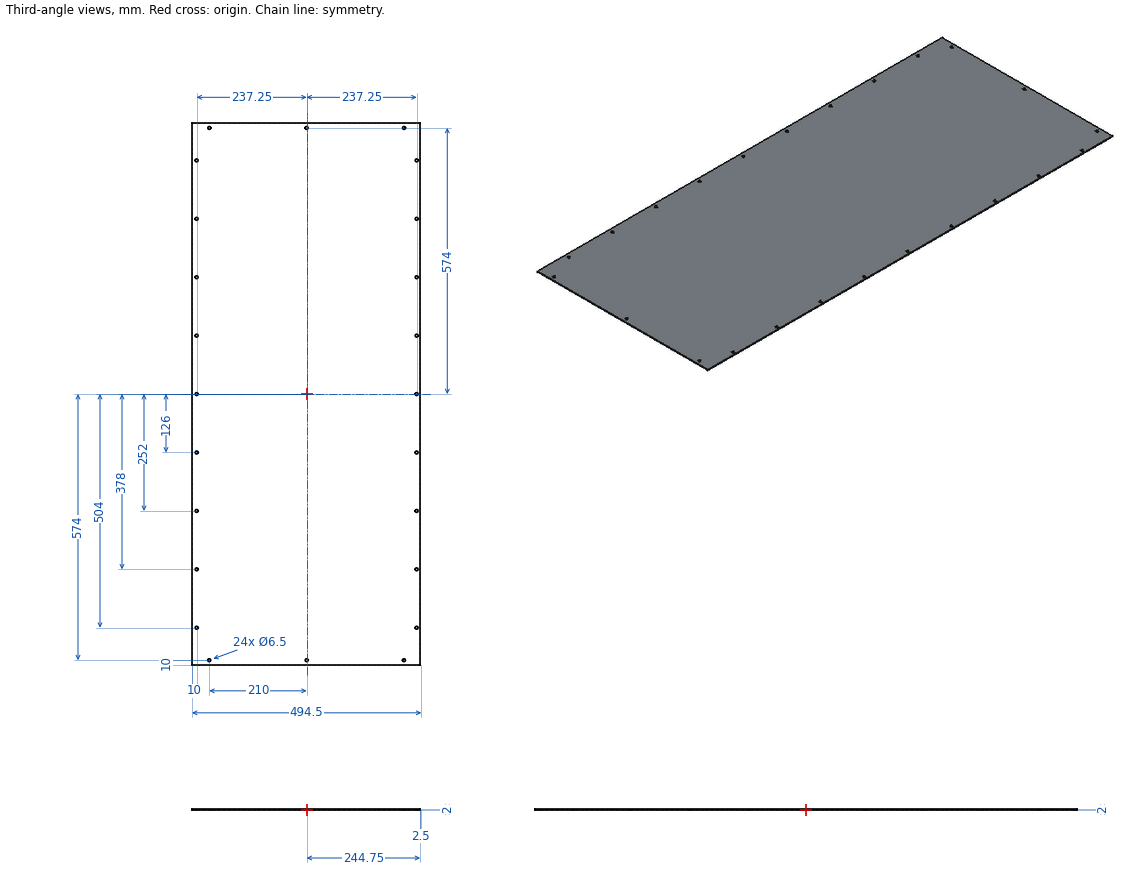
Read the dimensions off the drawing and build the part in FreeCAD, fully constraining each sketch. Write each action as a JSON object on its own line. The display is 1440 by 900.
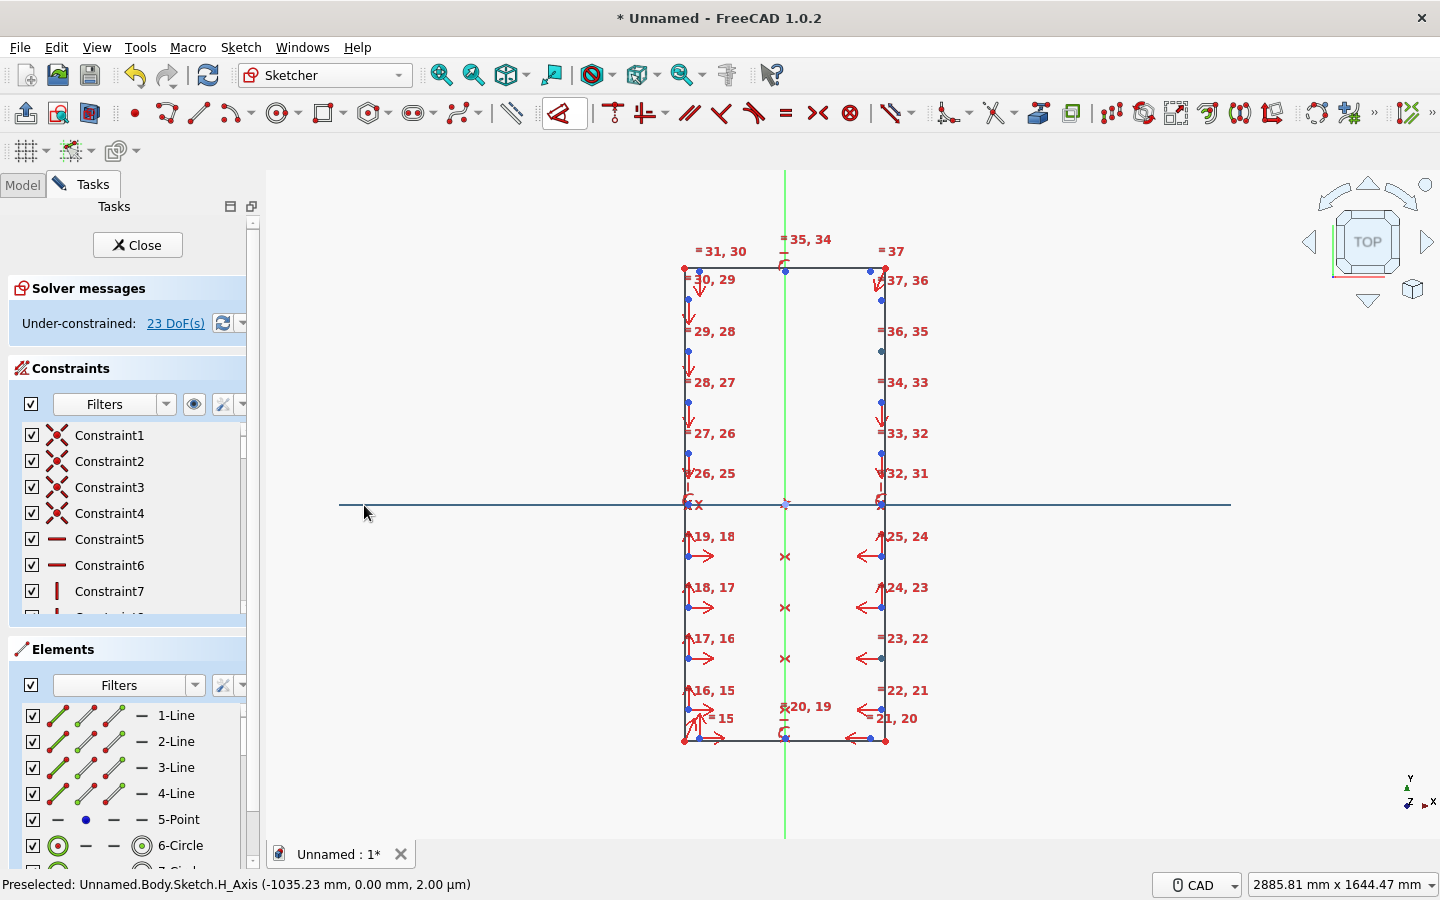
{"action": "key", "text": "s"}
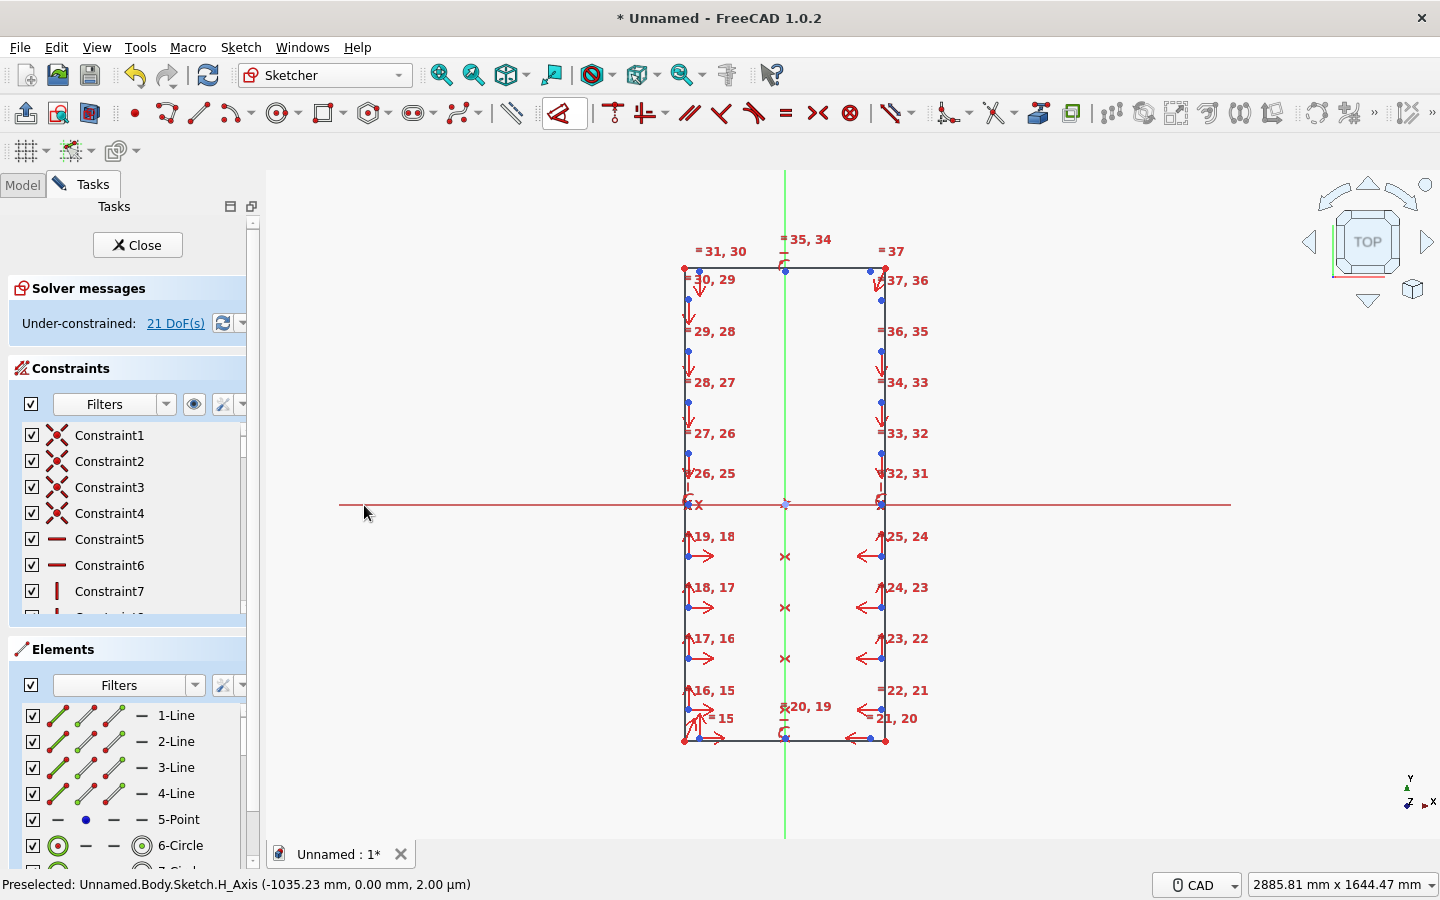
{"action": "left_click", "coordinate": [882, 710]}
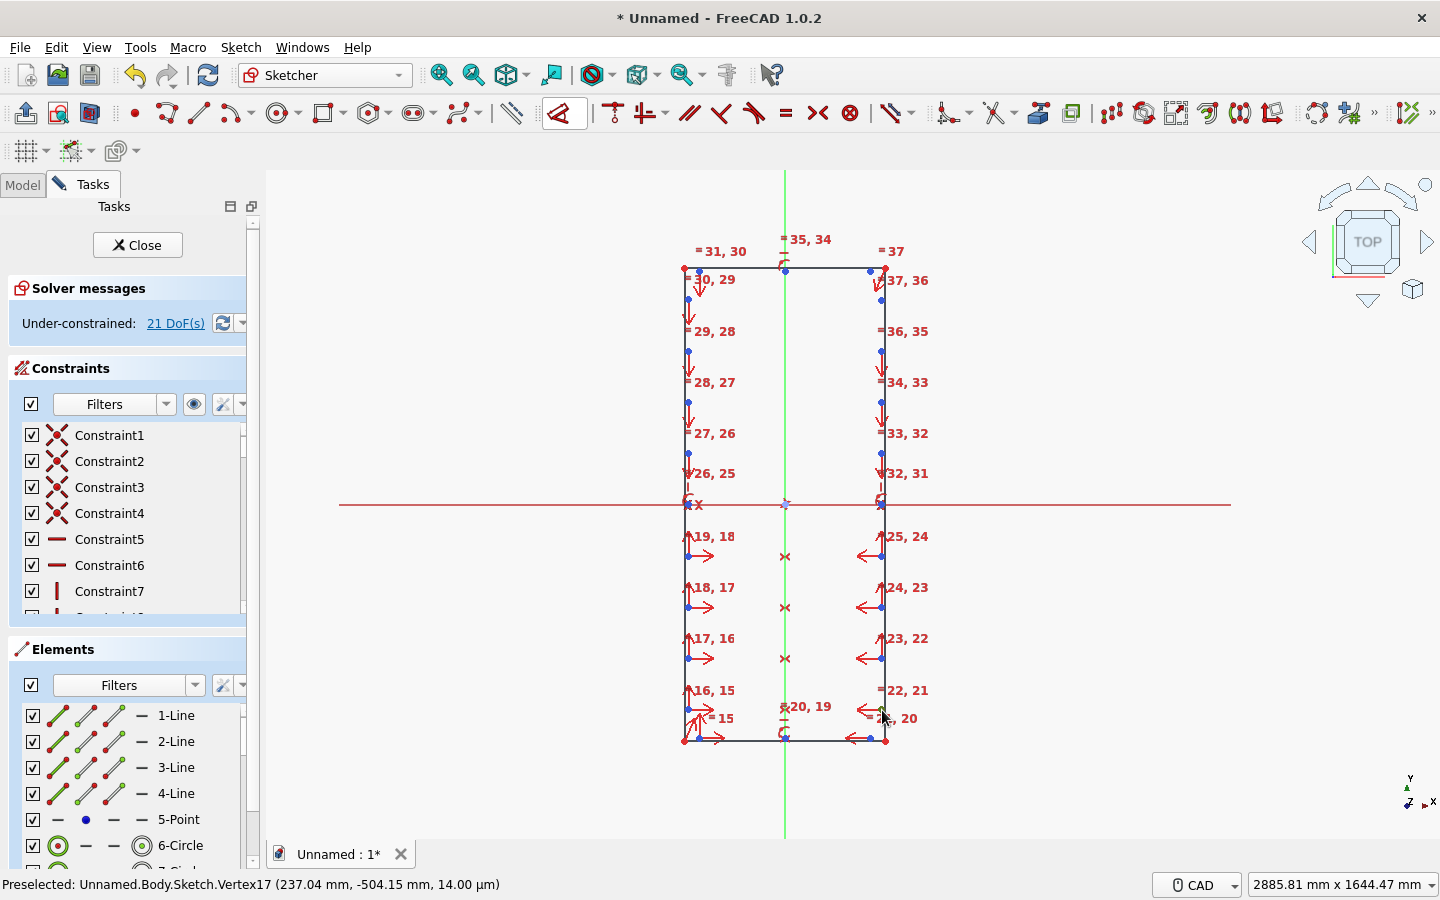
{"action": "left_click", "coordinate": [882, 300]}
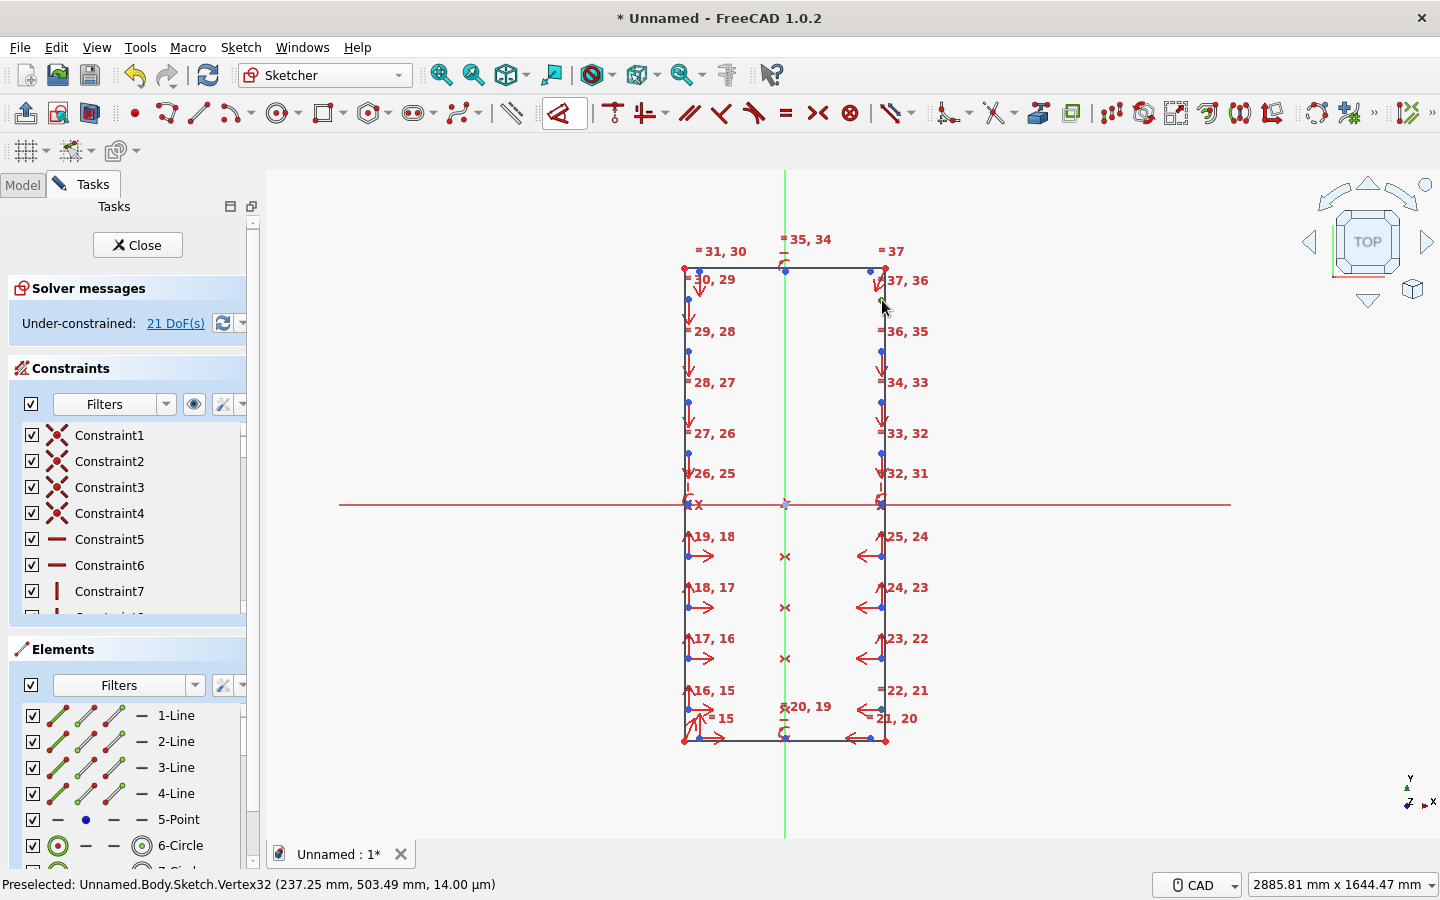
{"action": "left_click", "coordinate": [364, 505]}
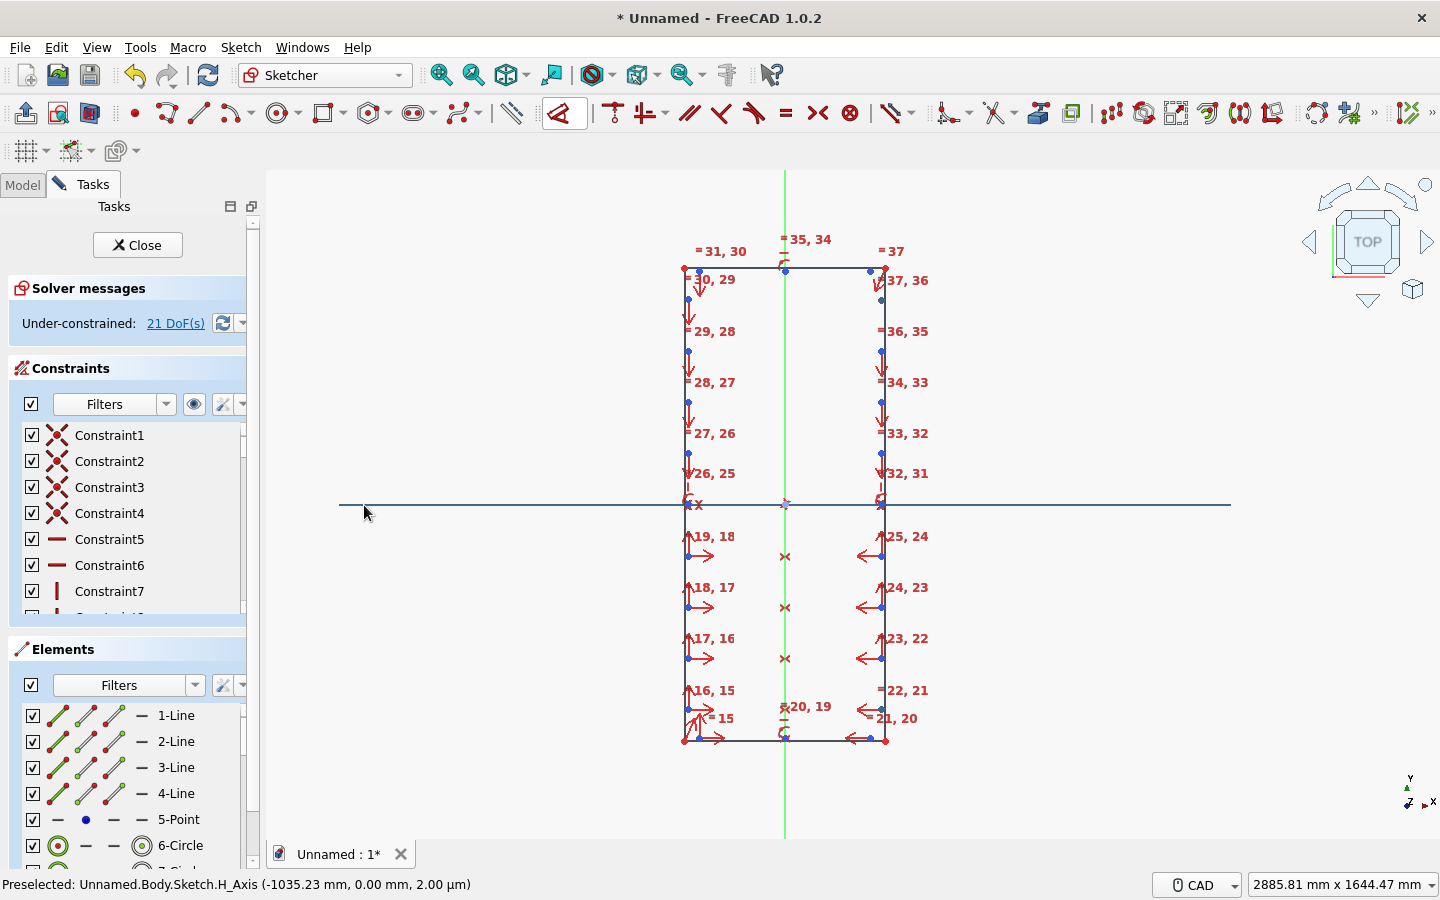
{"action": "key", "text": "s"}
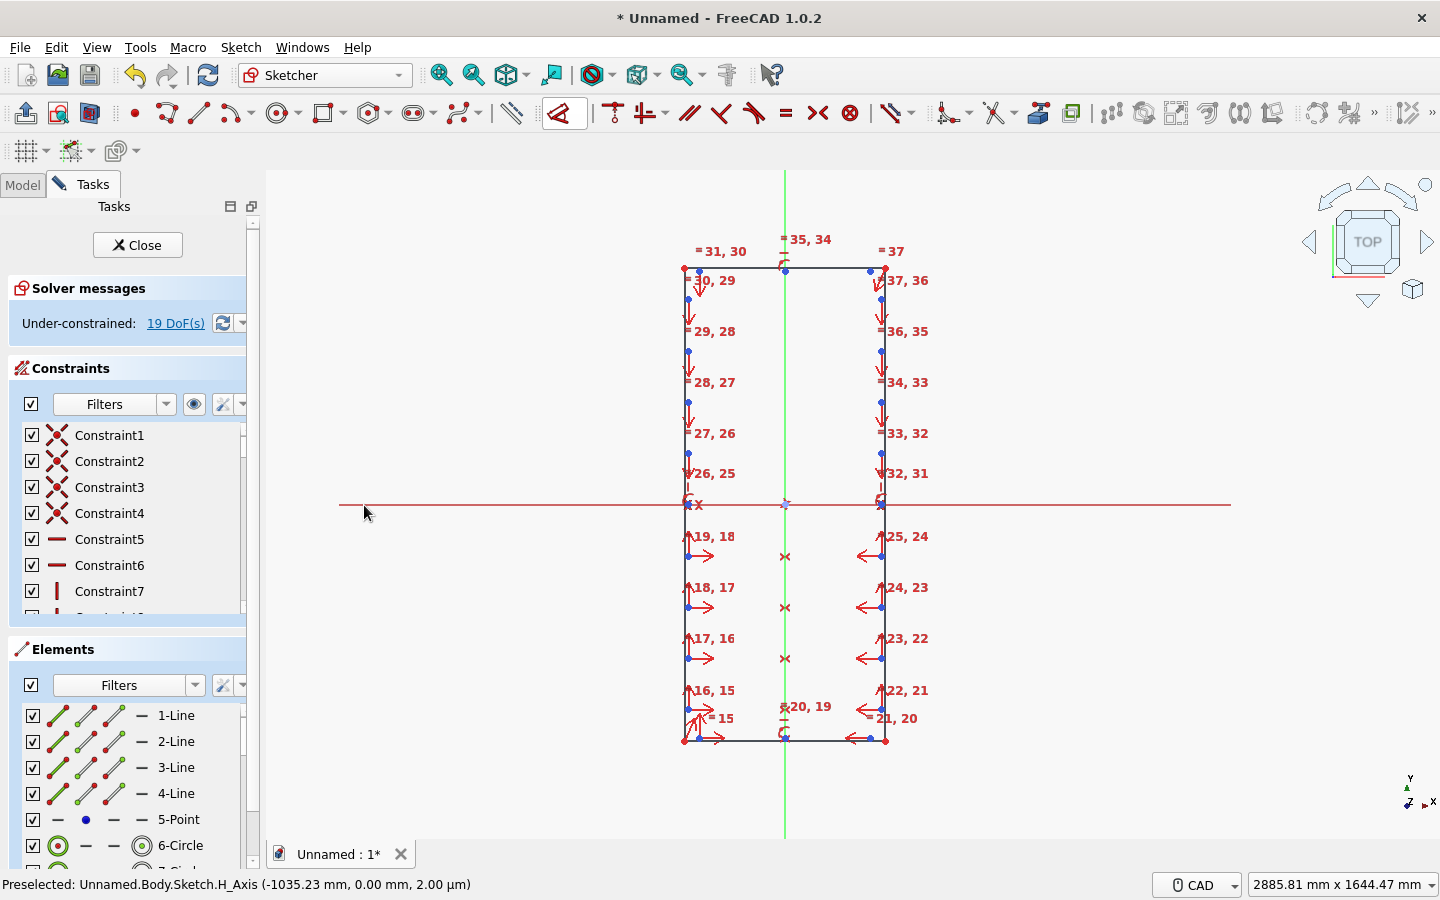
{"action": "left_click", "coordinate": [871, 738]}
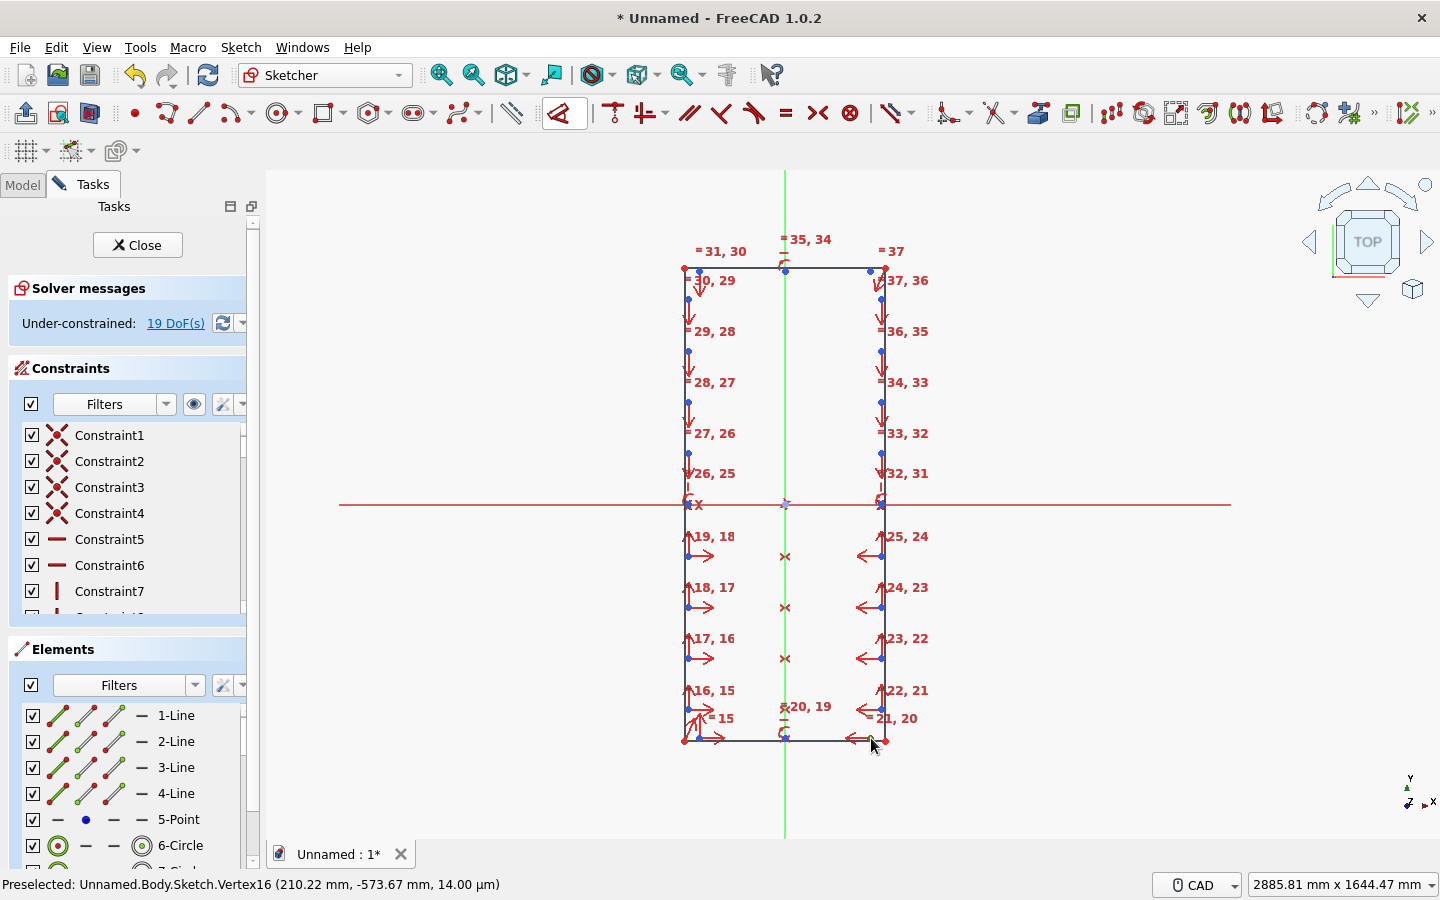
{"action": "left_click", "coordinate": [870, 272]}